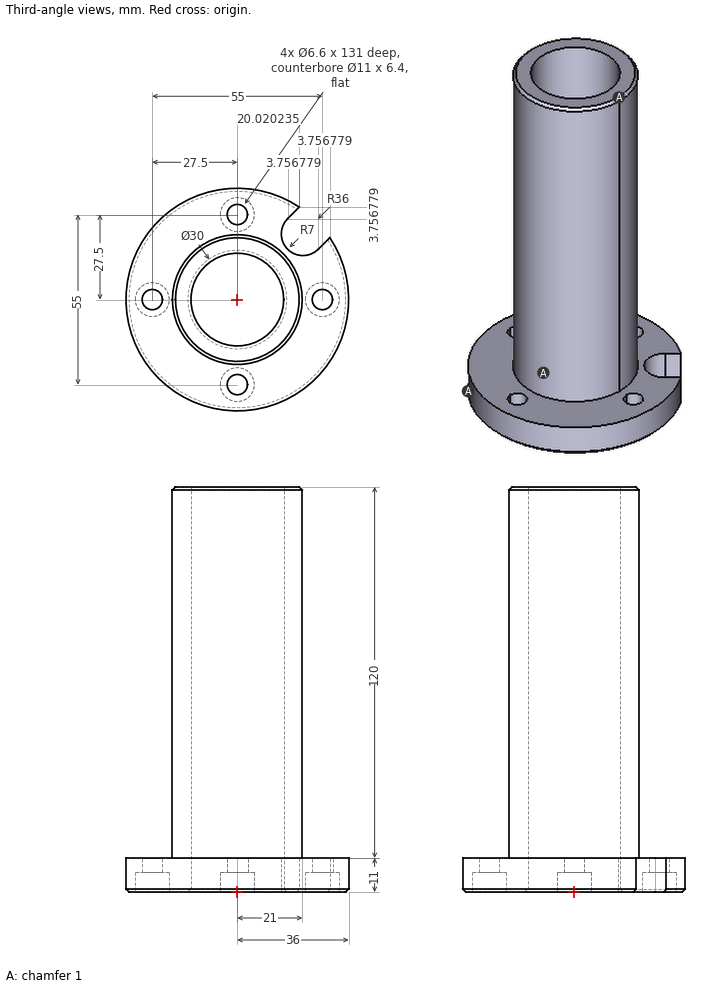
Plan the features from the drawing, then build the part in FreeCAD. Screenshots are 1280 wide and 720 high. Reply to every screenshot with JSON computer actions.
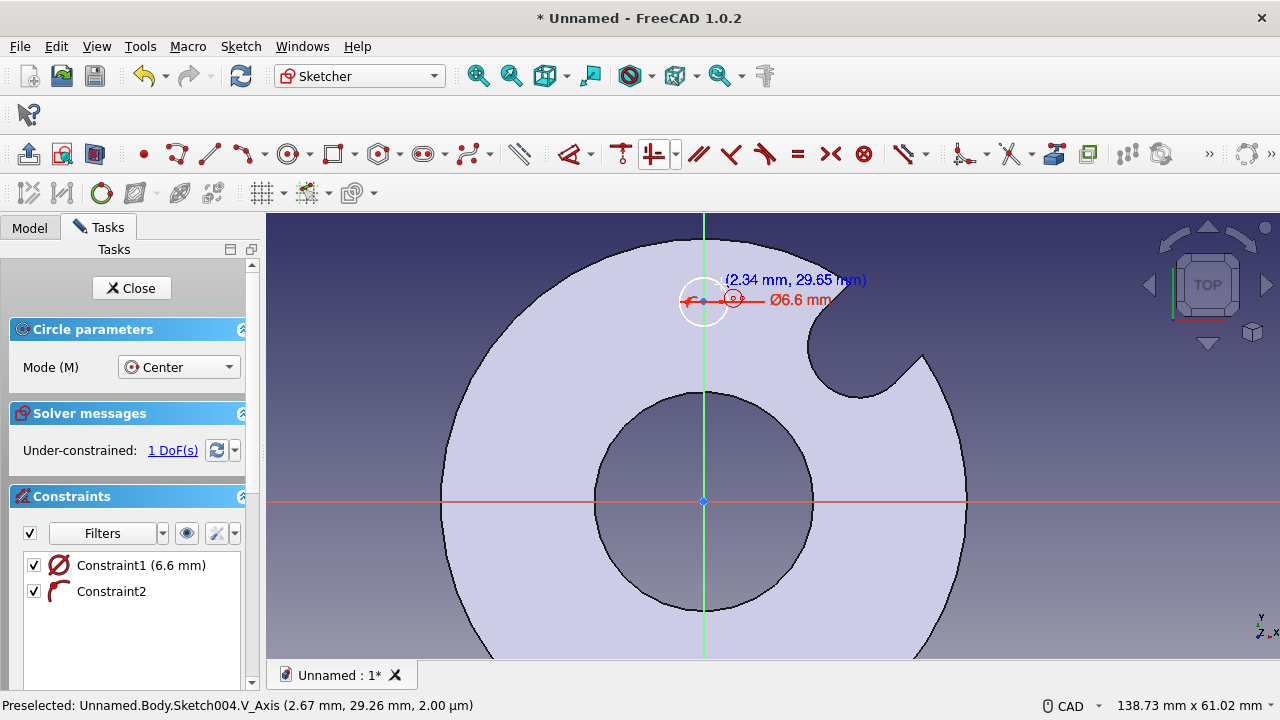
{"action": "left_click", "coordinate": [503, 502]}
{"action": "mouse_move", "coordinate": [520, 485]}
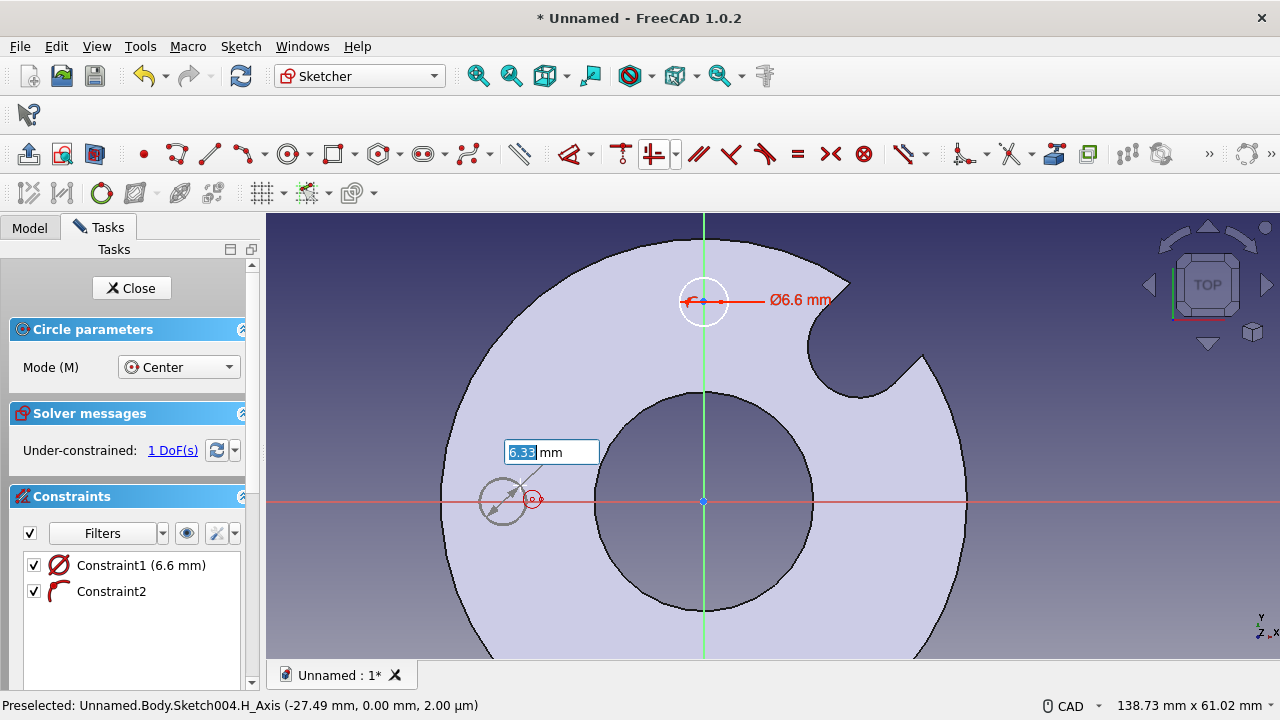
{"action": "type", "text": "6.6"}
{"action": "key", "text": "Return"}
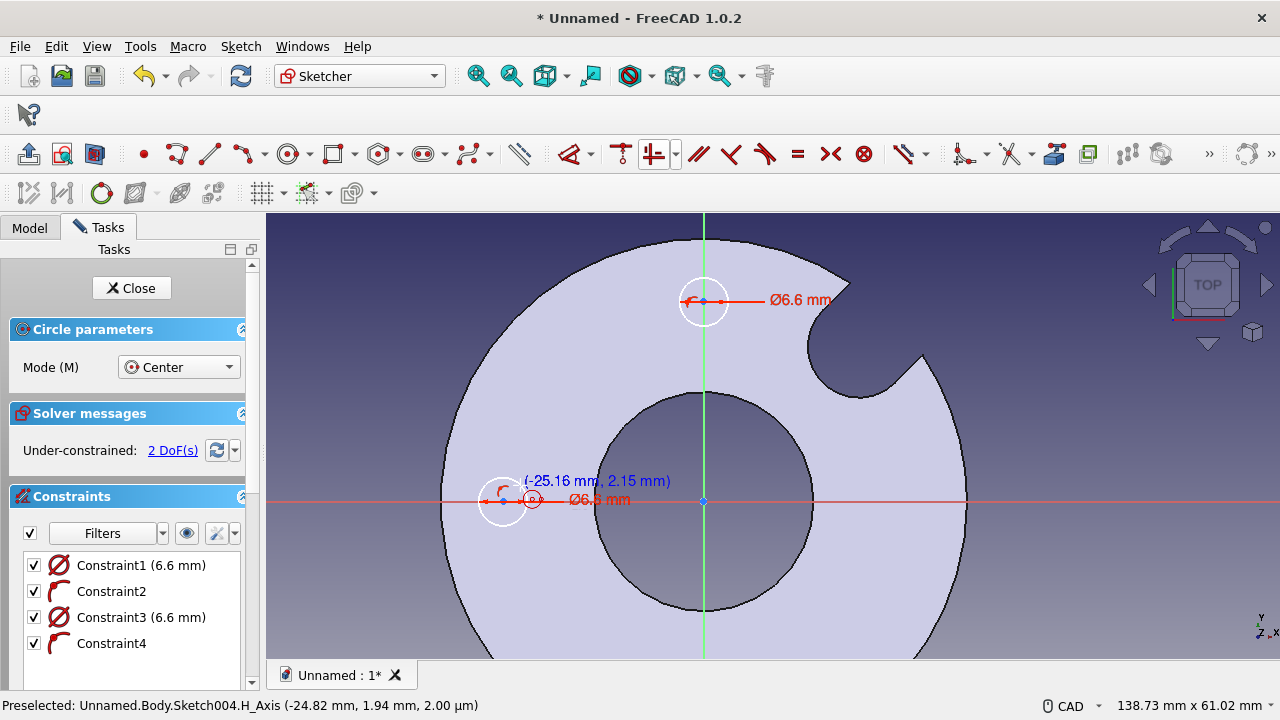
{"action": "scroll", "coordinate": [706, 302], "scroll_direction": "down", "scroll_amount": 2}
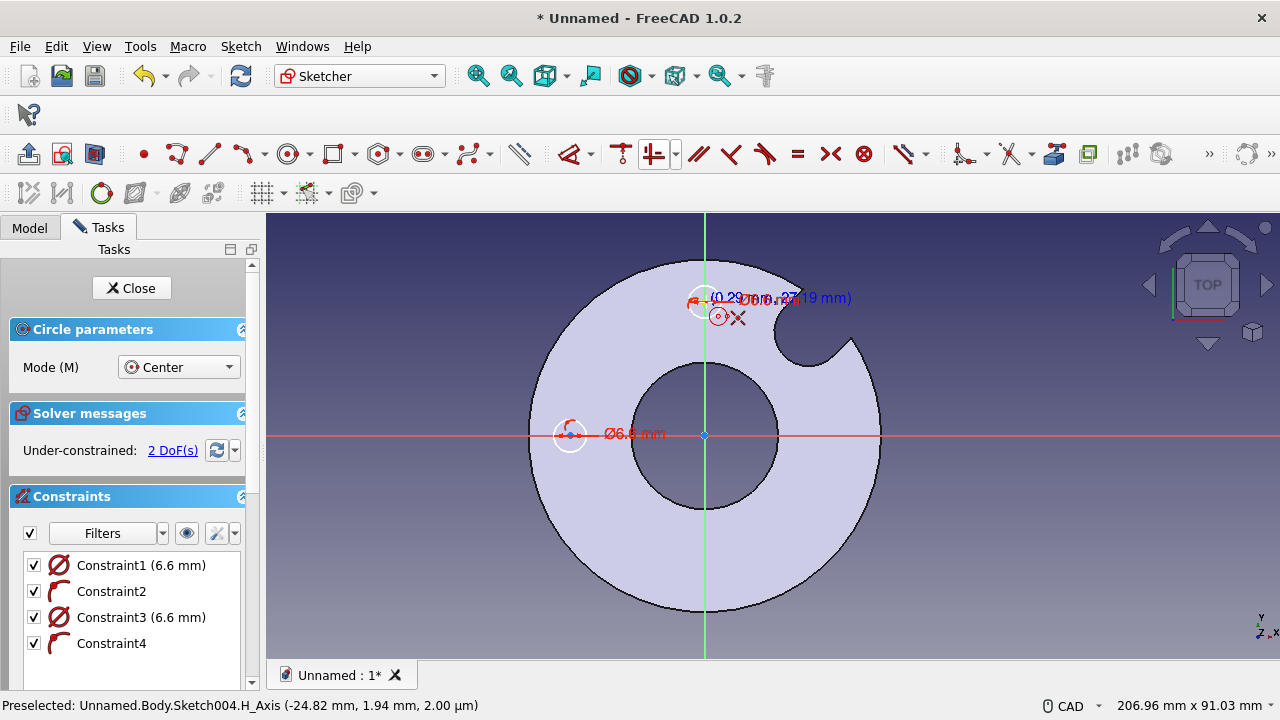
{"action": "scroll", "coordinate": [705, 571], "scroll_direction": "up", "scroll_amount": 2}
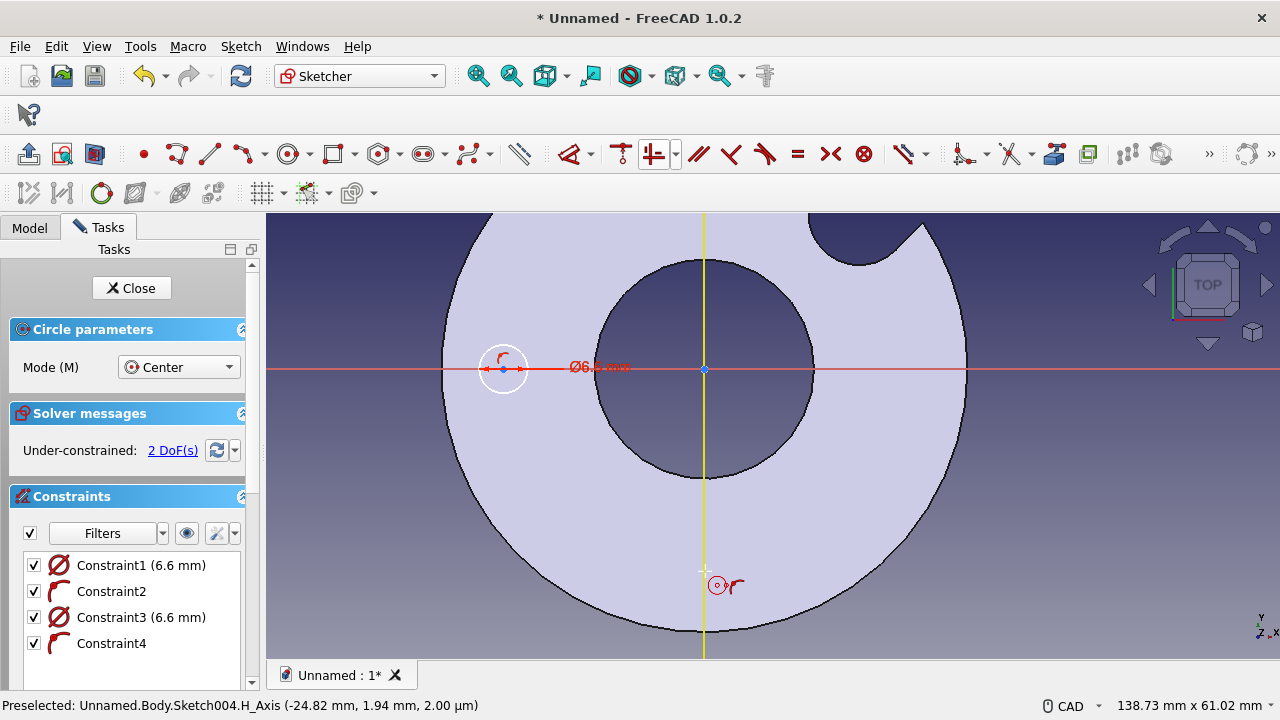
{"action": "left_click", "coordinate": [704, 570]}
{"action": "mouse_move", "coordinate": [721, 553]}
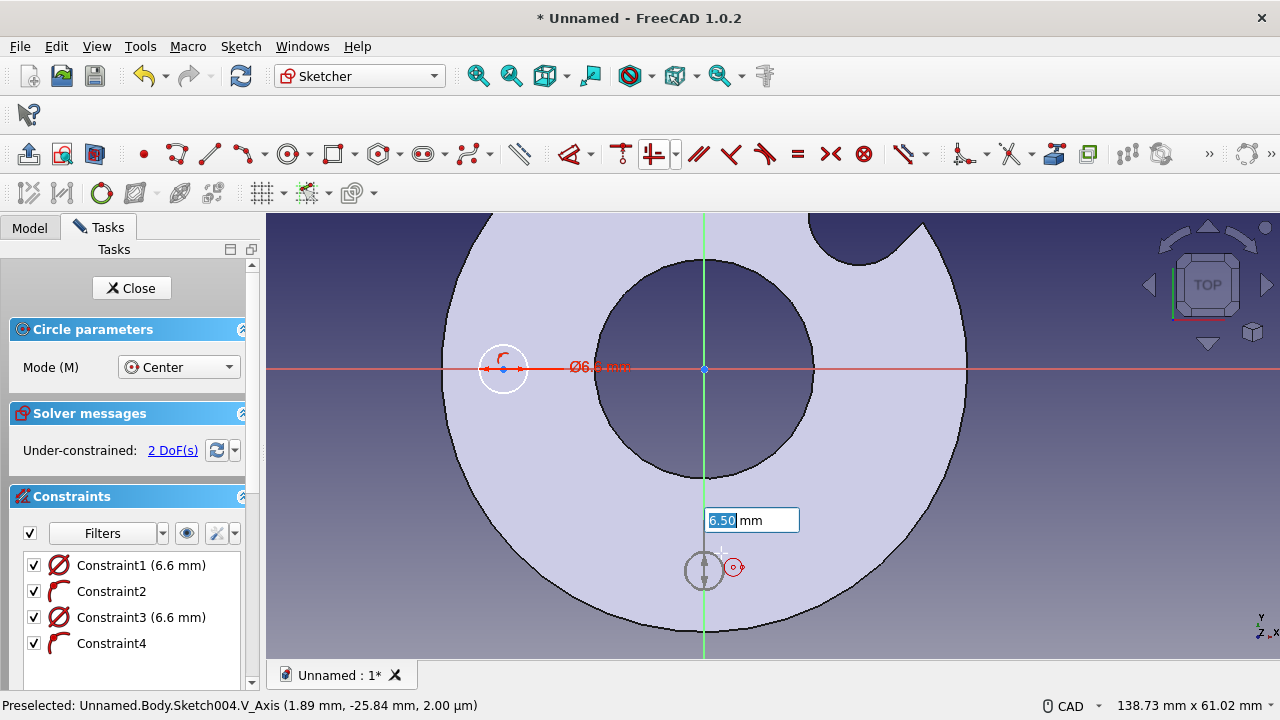
{"action": "type", "text": "6.6"}
{"action": "key", "text": "Return"}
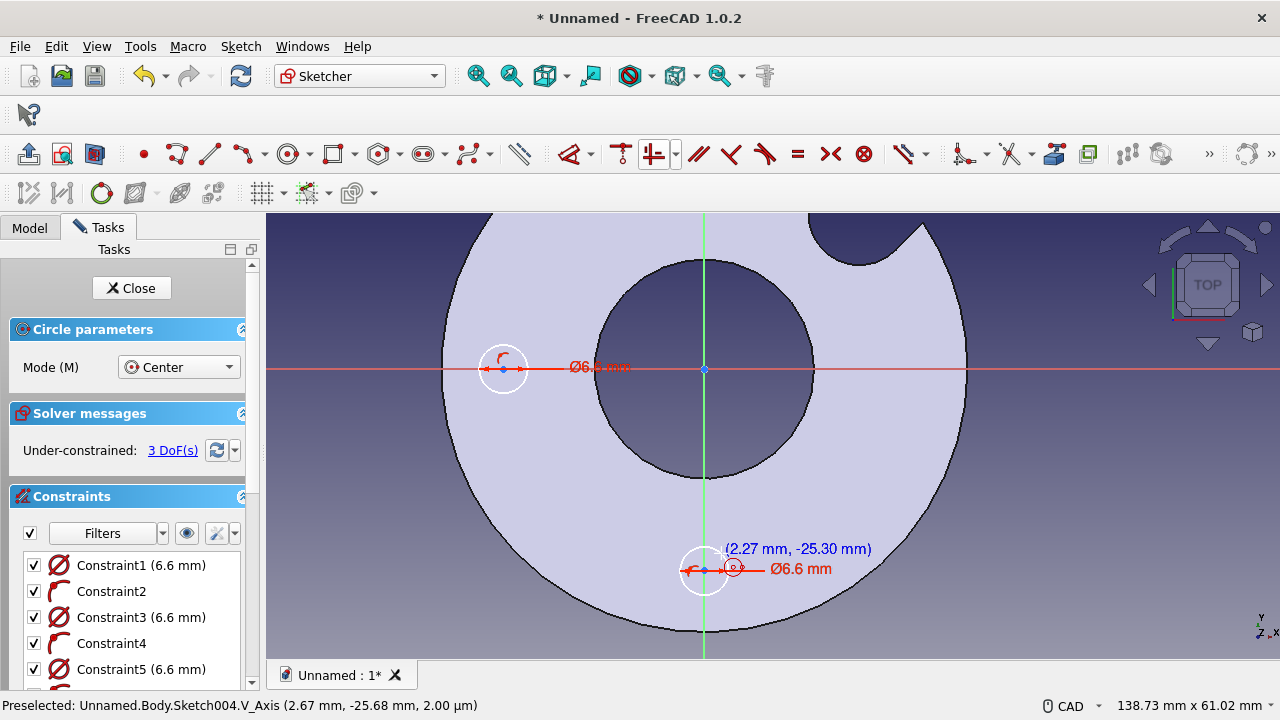
{"action": "left_click", "coordinate": [905, 369]}
{"action": "mouse_move", "coordinate": [922, 352]}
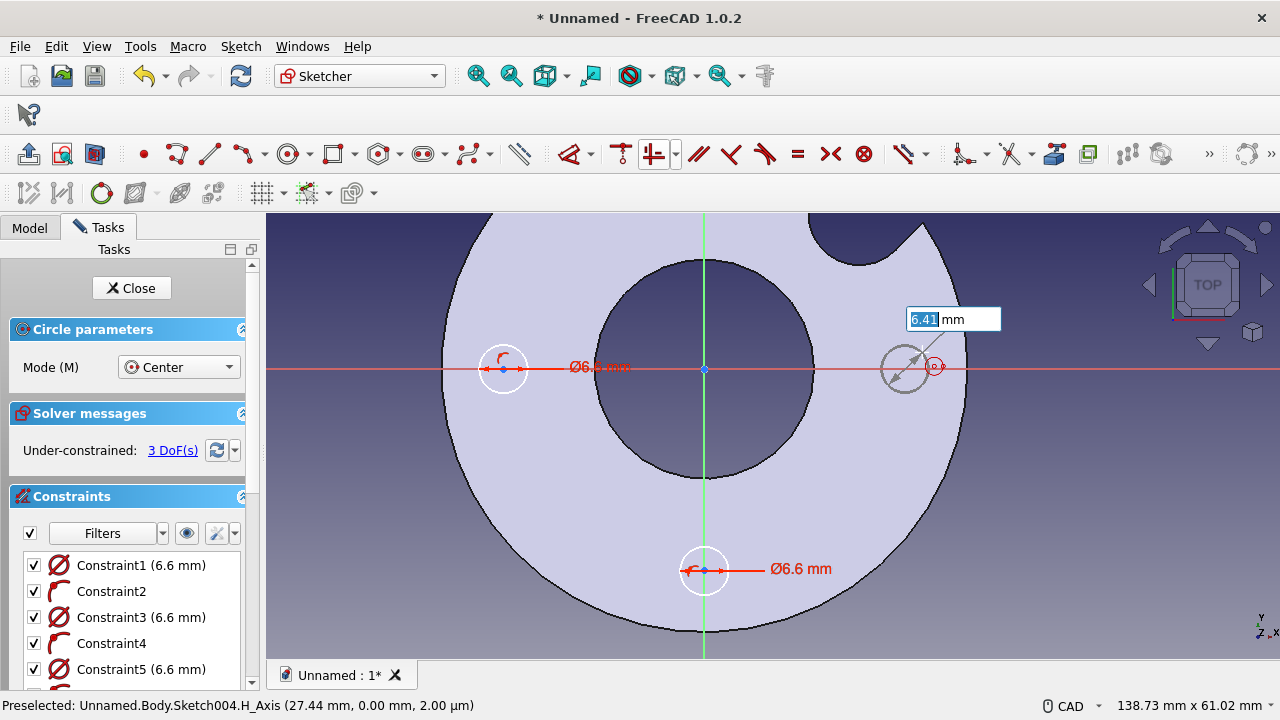
{"action": "type", "text": "6.6"}
{"action": "key", "text": "Return"}
{"action": "key", "text": "Escape"}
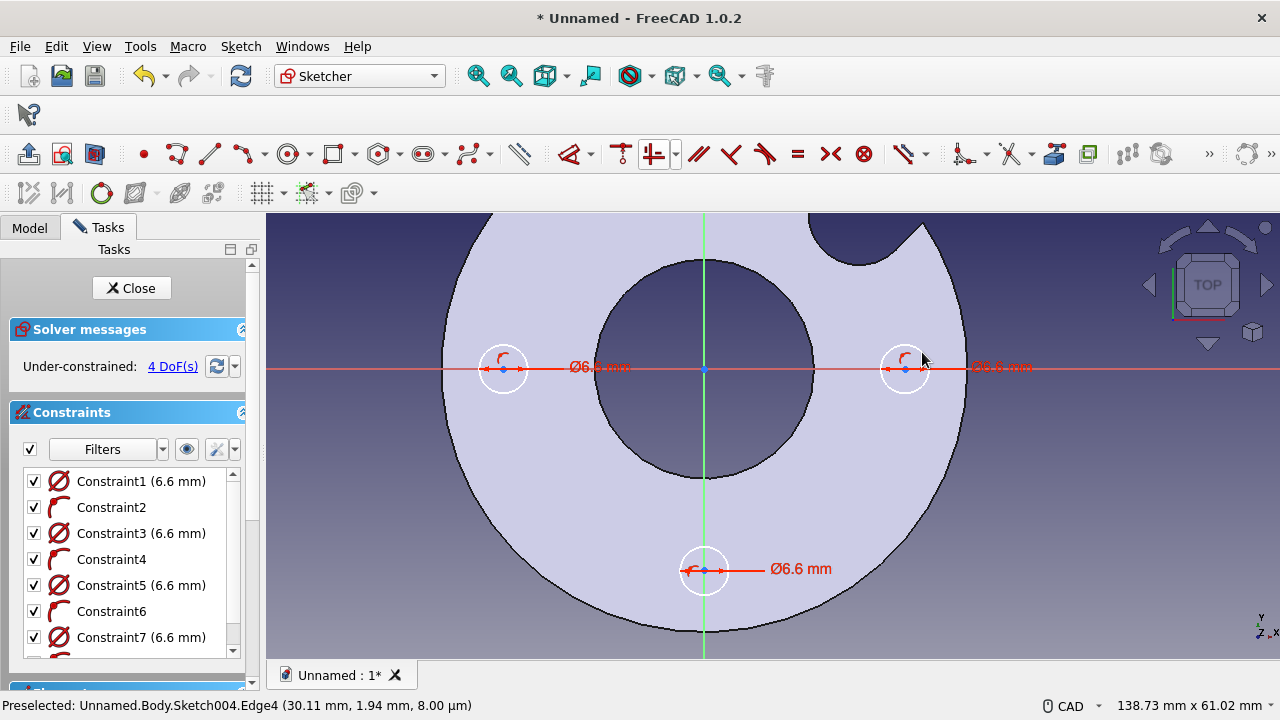
{"action": "key", "text": "d"}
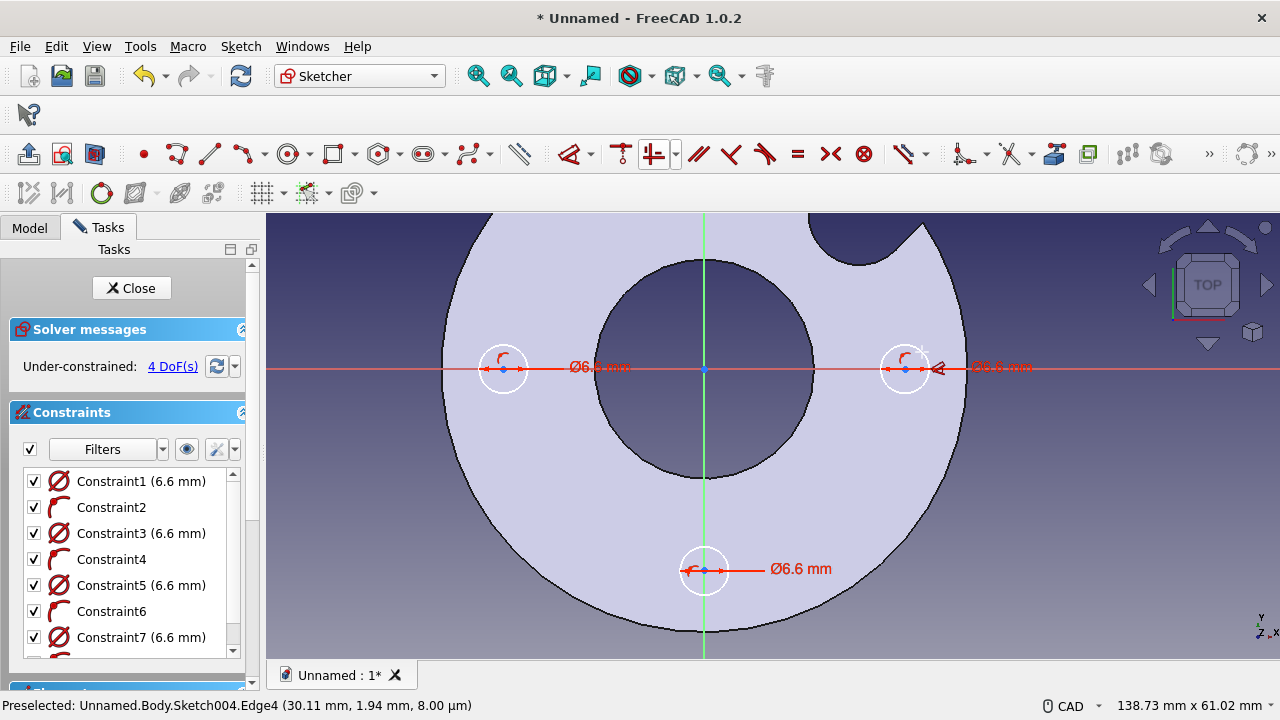
{"action": "scroll", "coordinate": [705, 572], "scroll_direction": "down", "scroll_amount": 2}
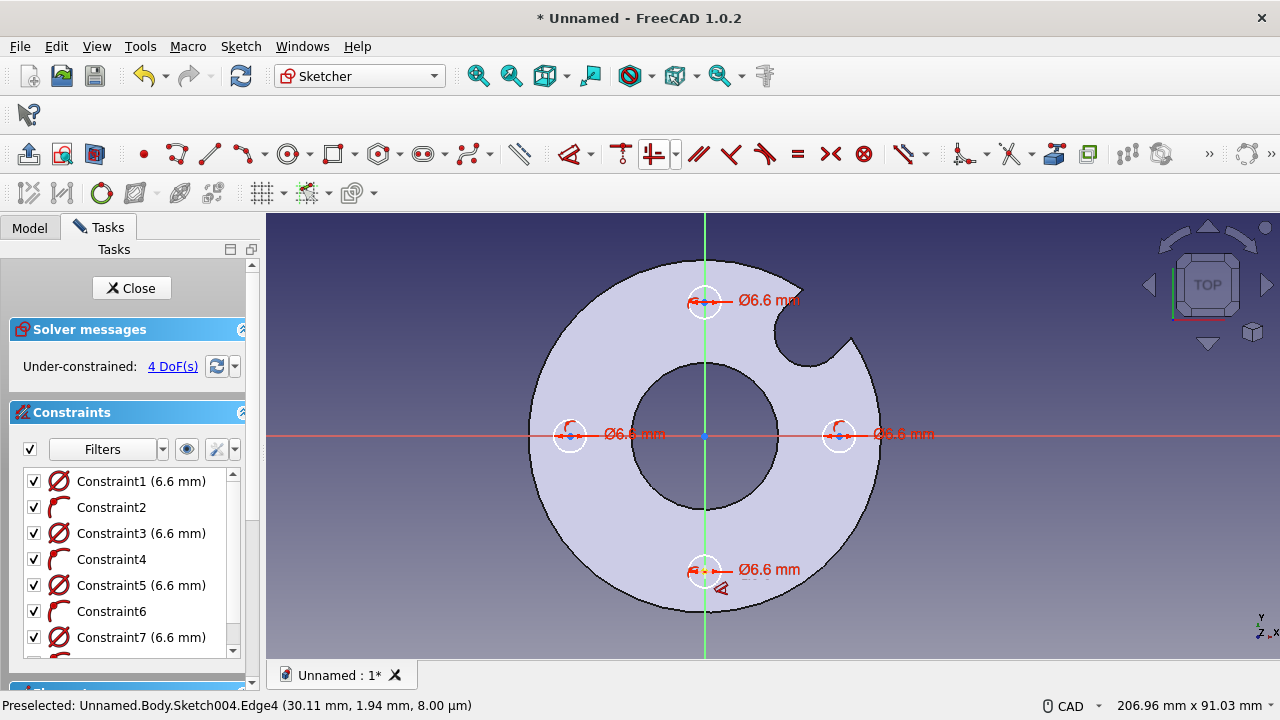
{"action": "left_click", "coordinate": [705, 302]}